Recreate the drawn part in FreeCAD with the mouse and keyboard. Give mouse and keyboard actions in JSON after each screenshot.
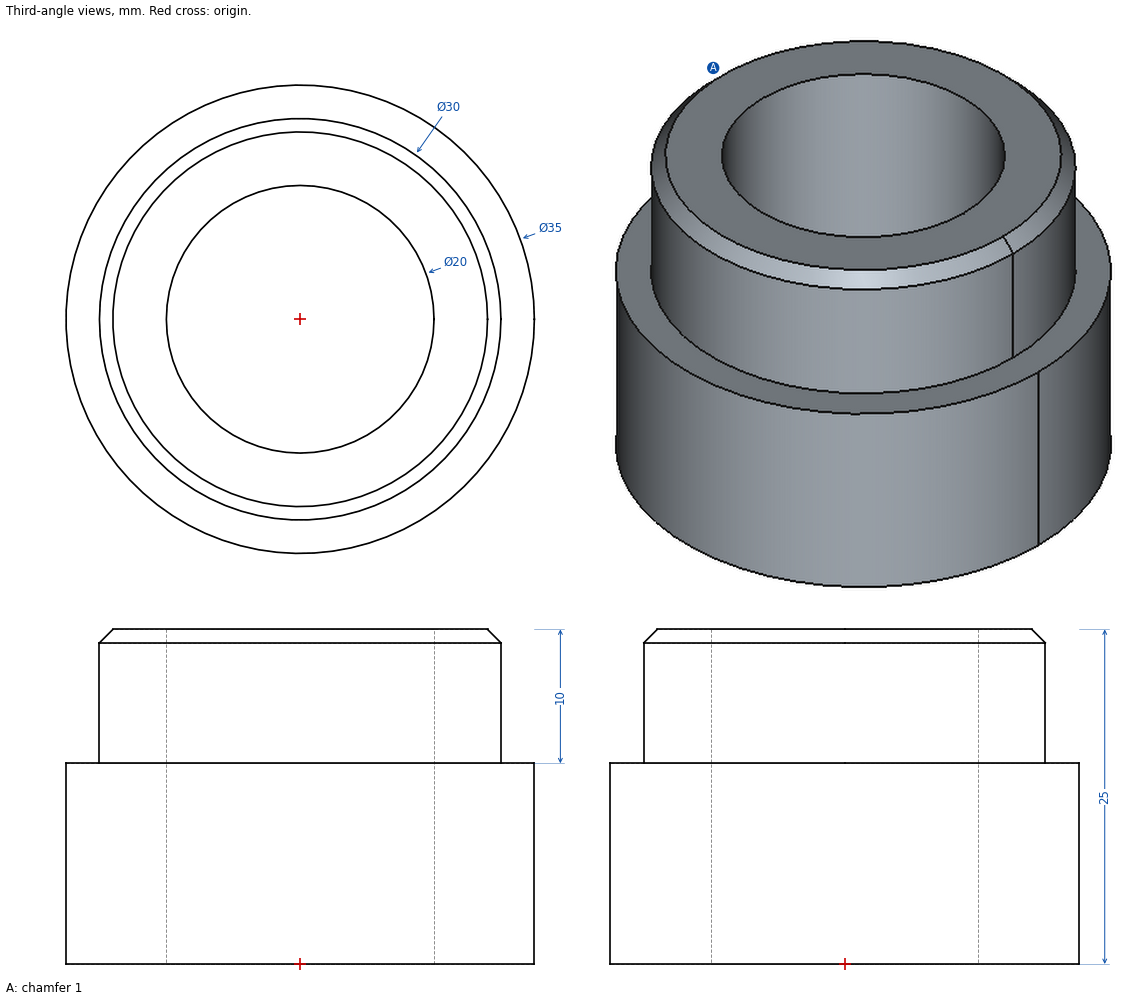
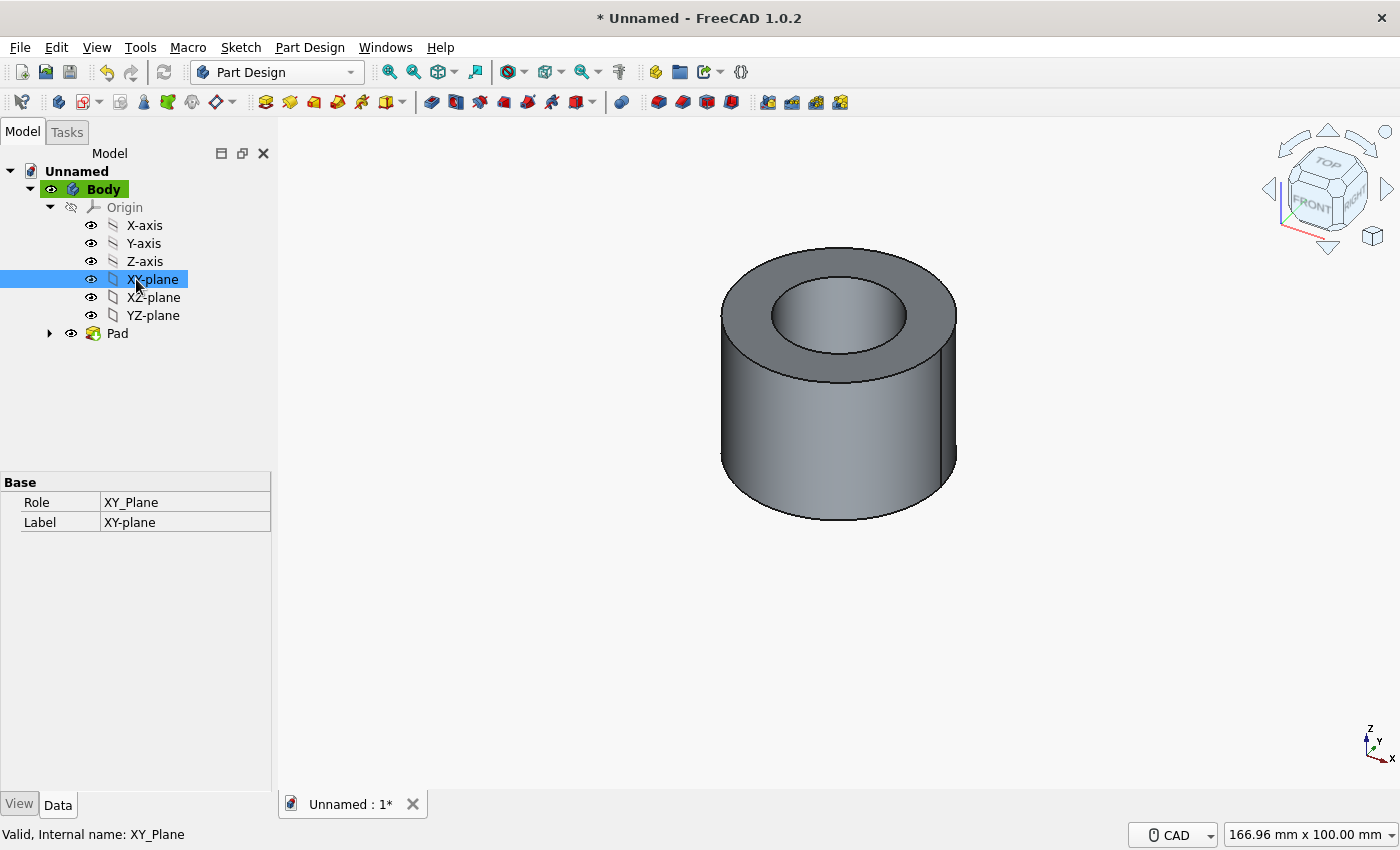
{"action": "left_click", "coordinate": [216, 102]}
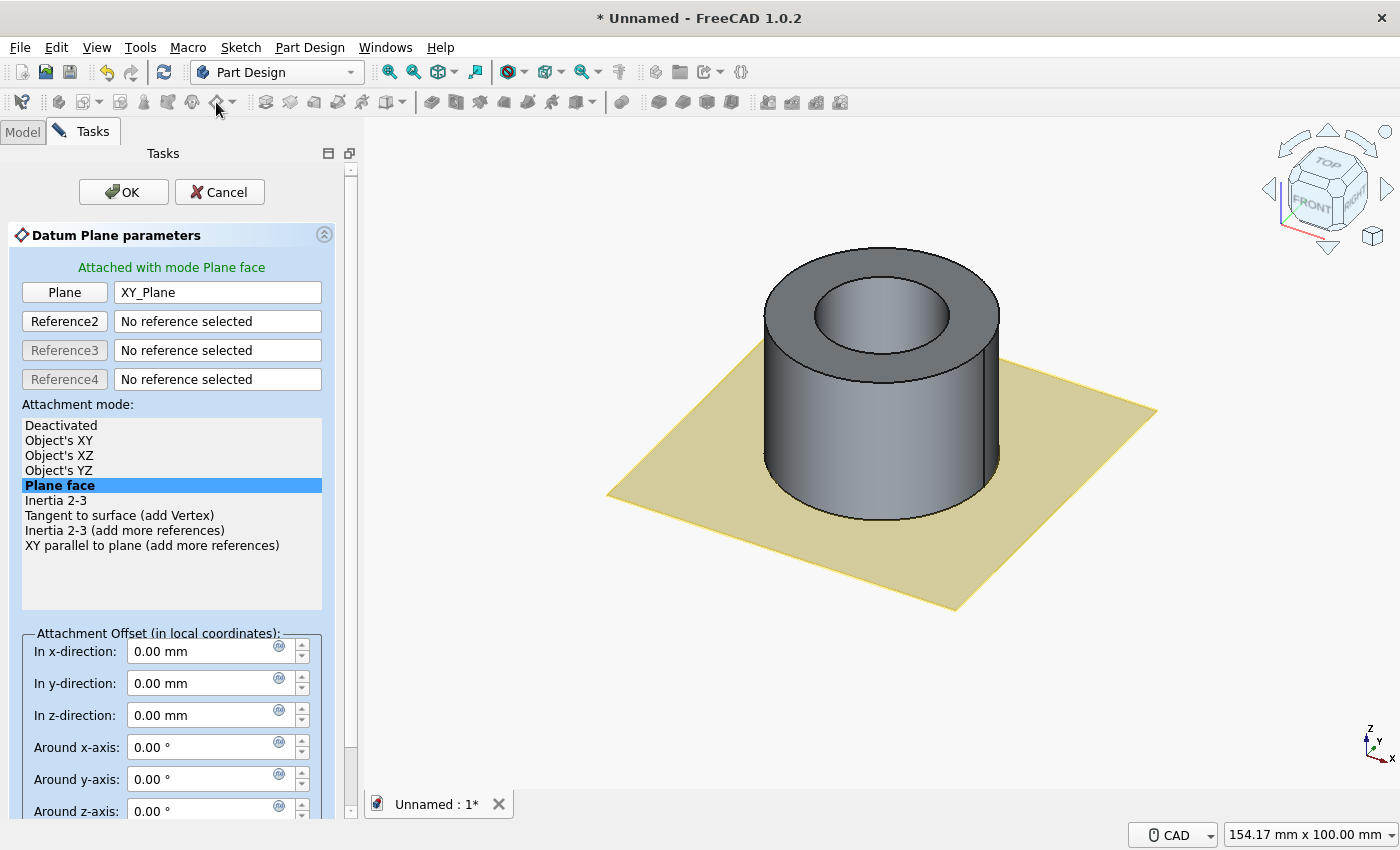
{"action": "triple_click", "coordinate": [210, 715]}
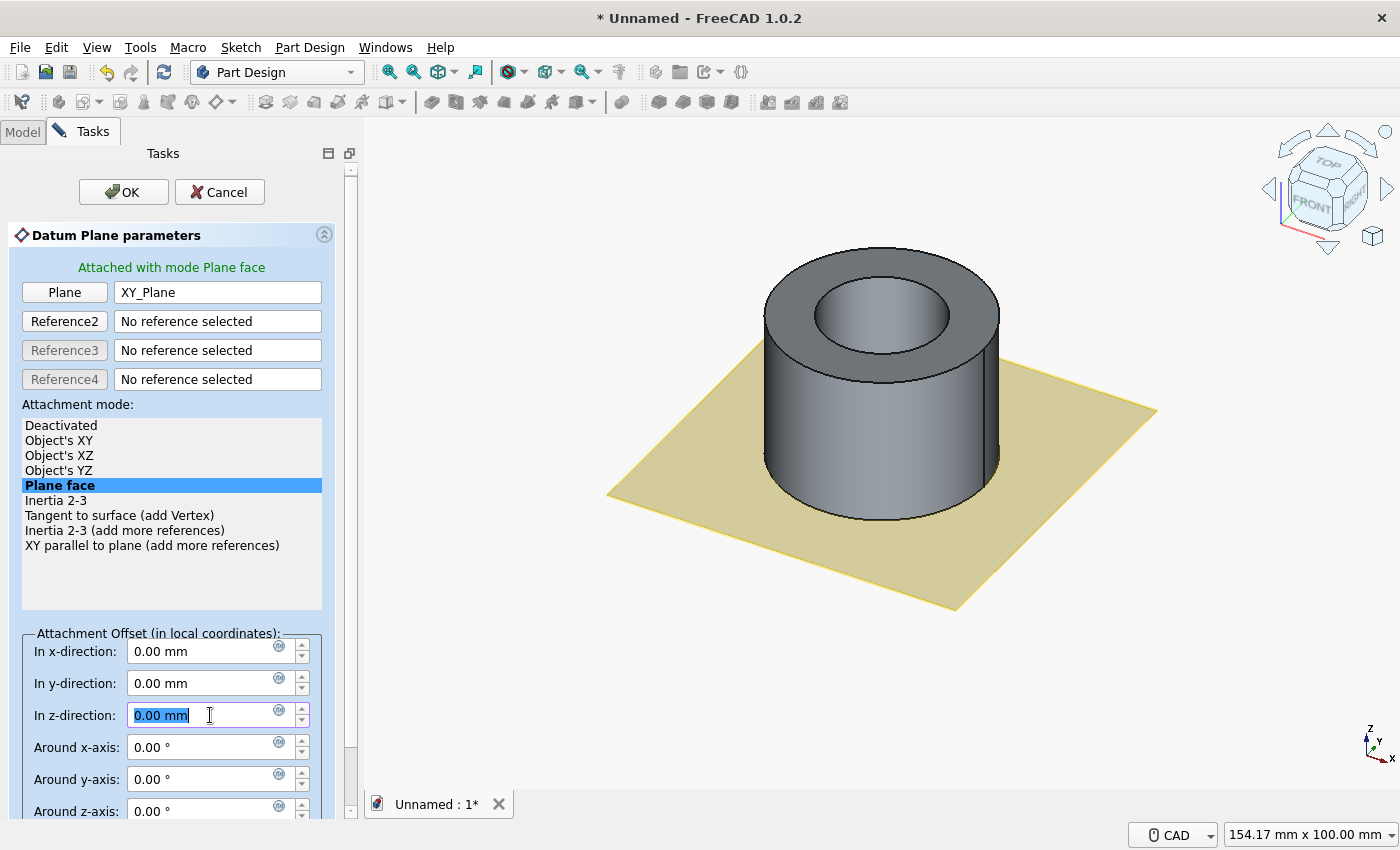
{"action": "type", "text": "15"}
{"action": "key", "text": "Tab"}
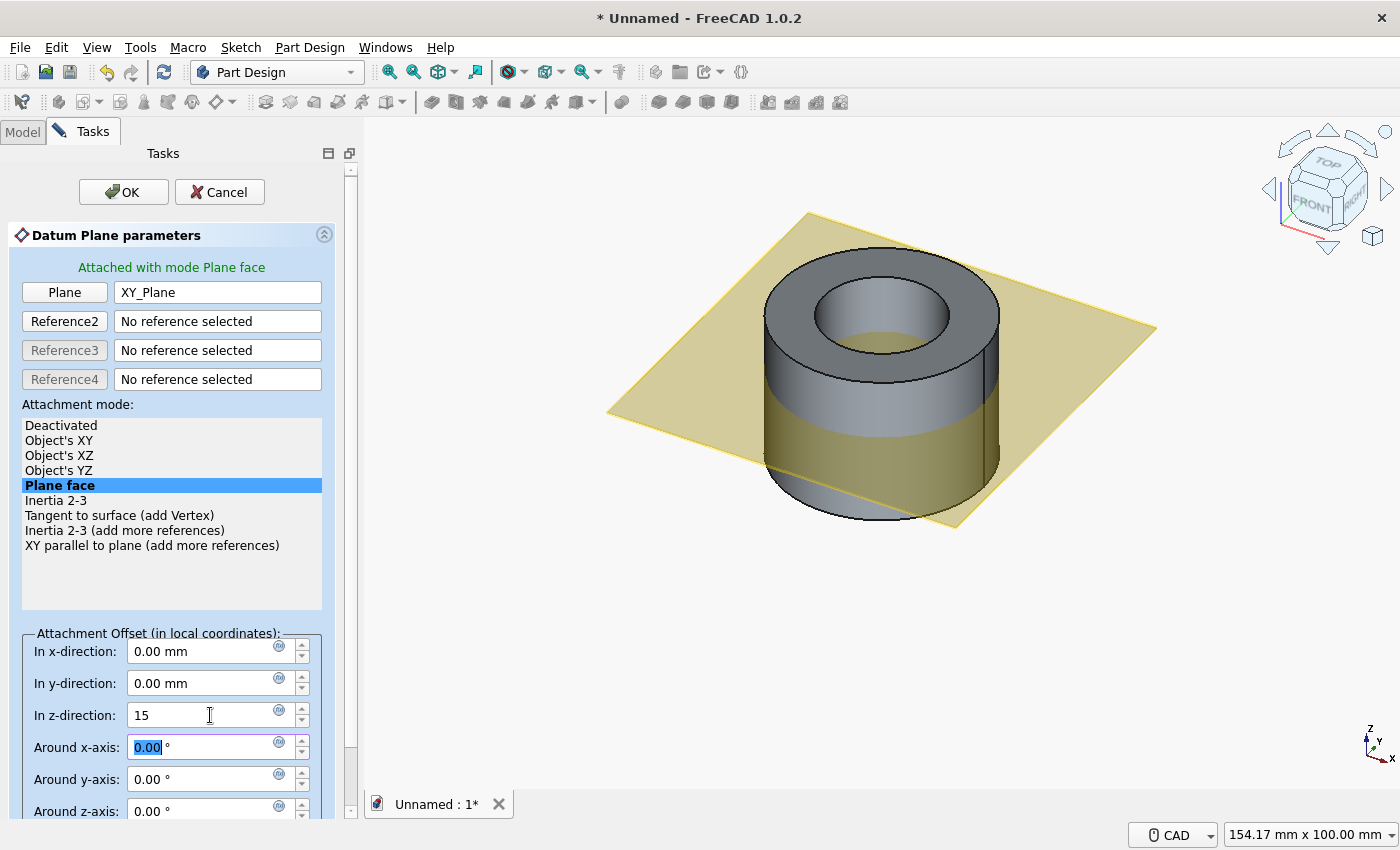
{"action": "left_click", "coordinate": [124, 192]}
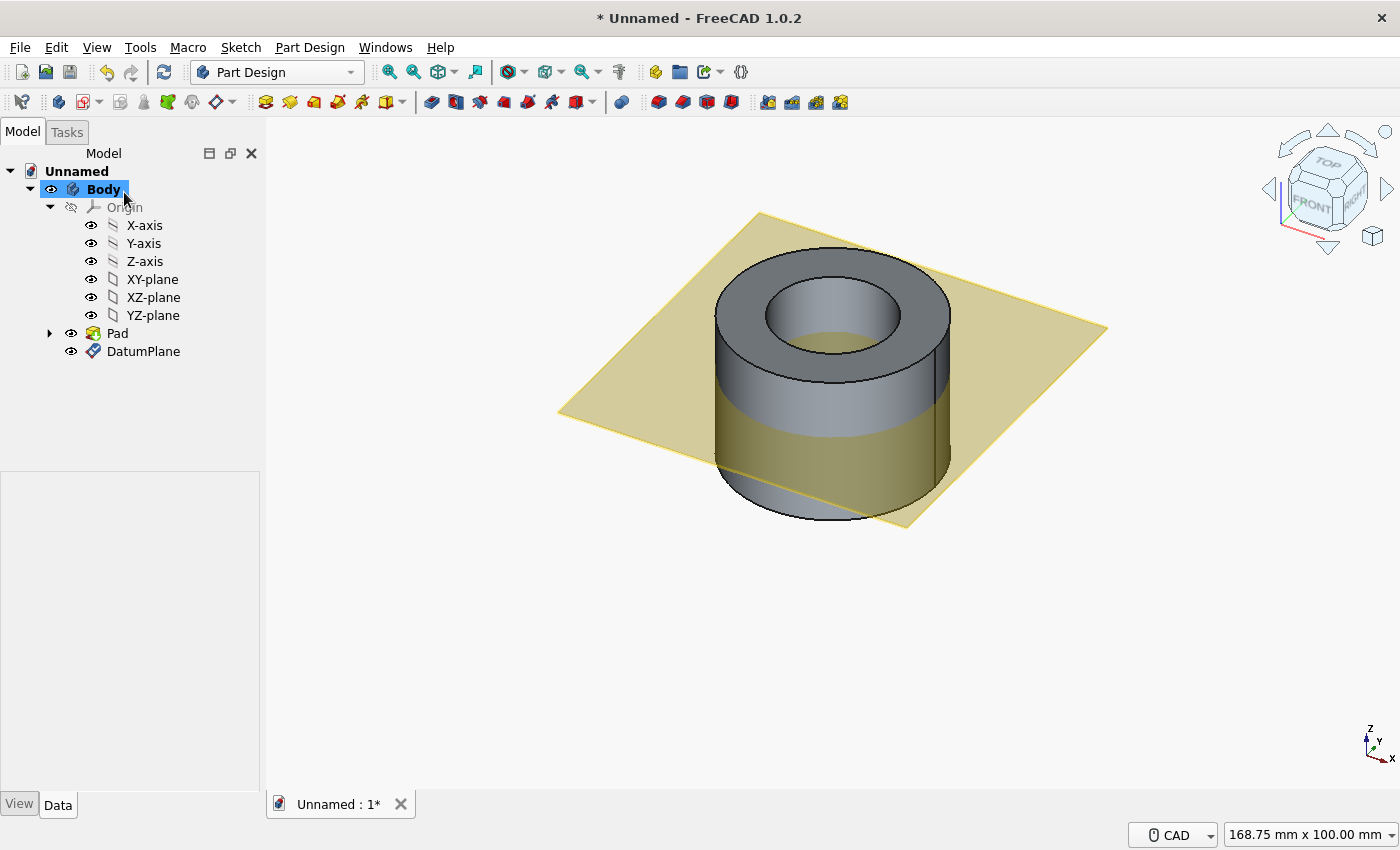
{"action": "left_click", "coordinate": [116, 351]}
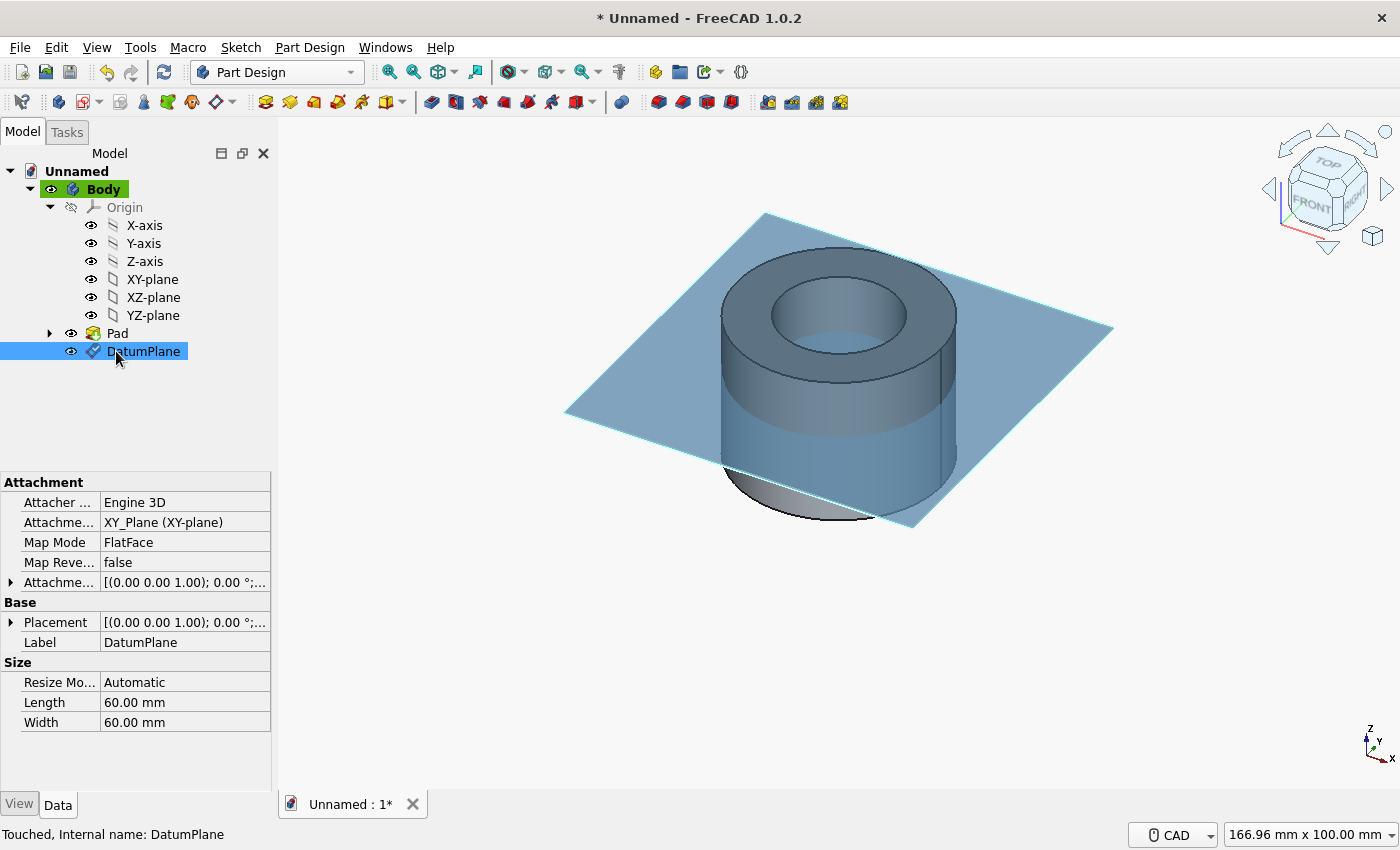
{"action": "left_click", "coordinate": [84, 102]}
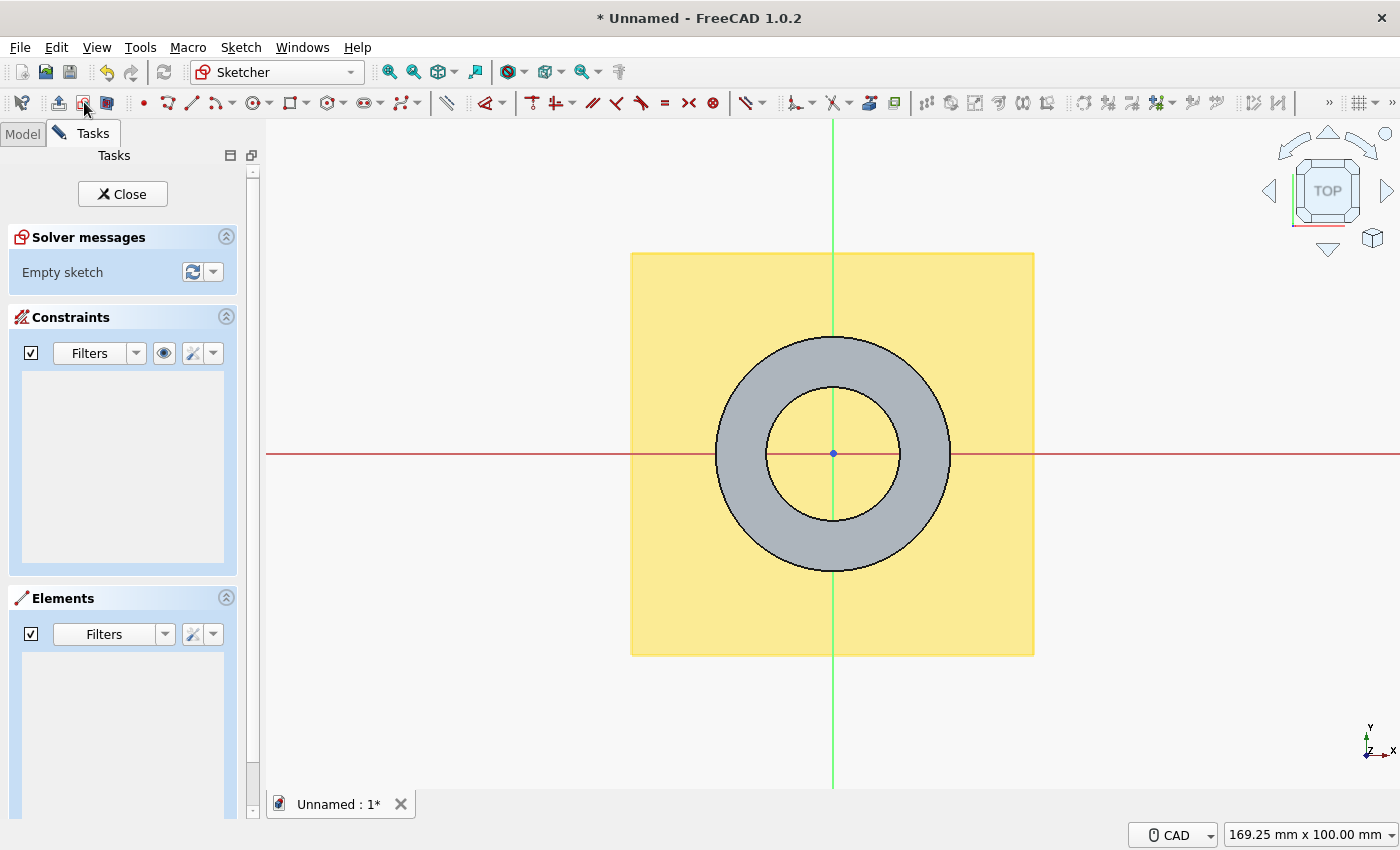
{"action": "left_click", "coordinate": [108, 104]}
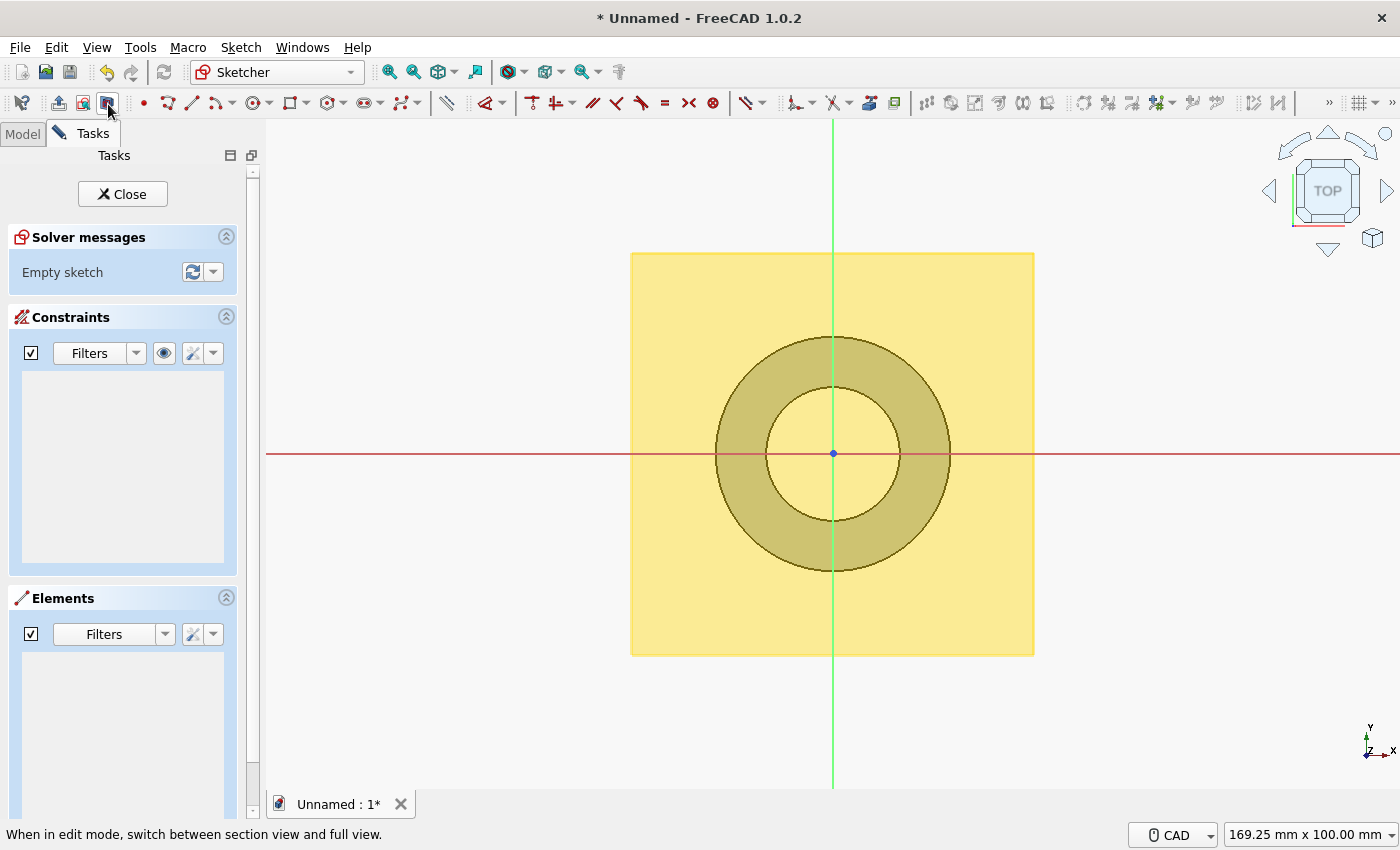
{"action": "scroll", "coordinate": [916, 454], "scroll_direction": "up", "scroll_amount": 3}